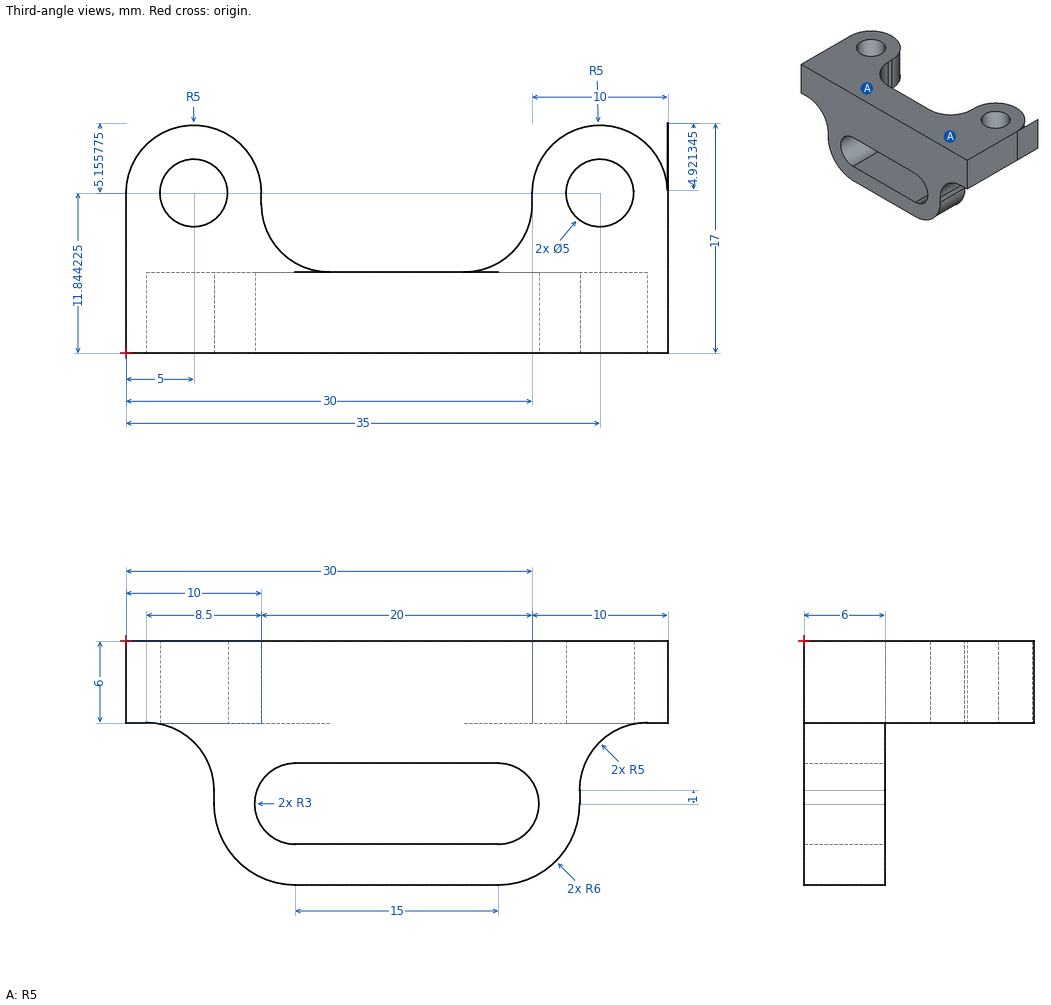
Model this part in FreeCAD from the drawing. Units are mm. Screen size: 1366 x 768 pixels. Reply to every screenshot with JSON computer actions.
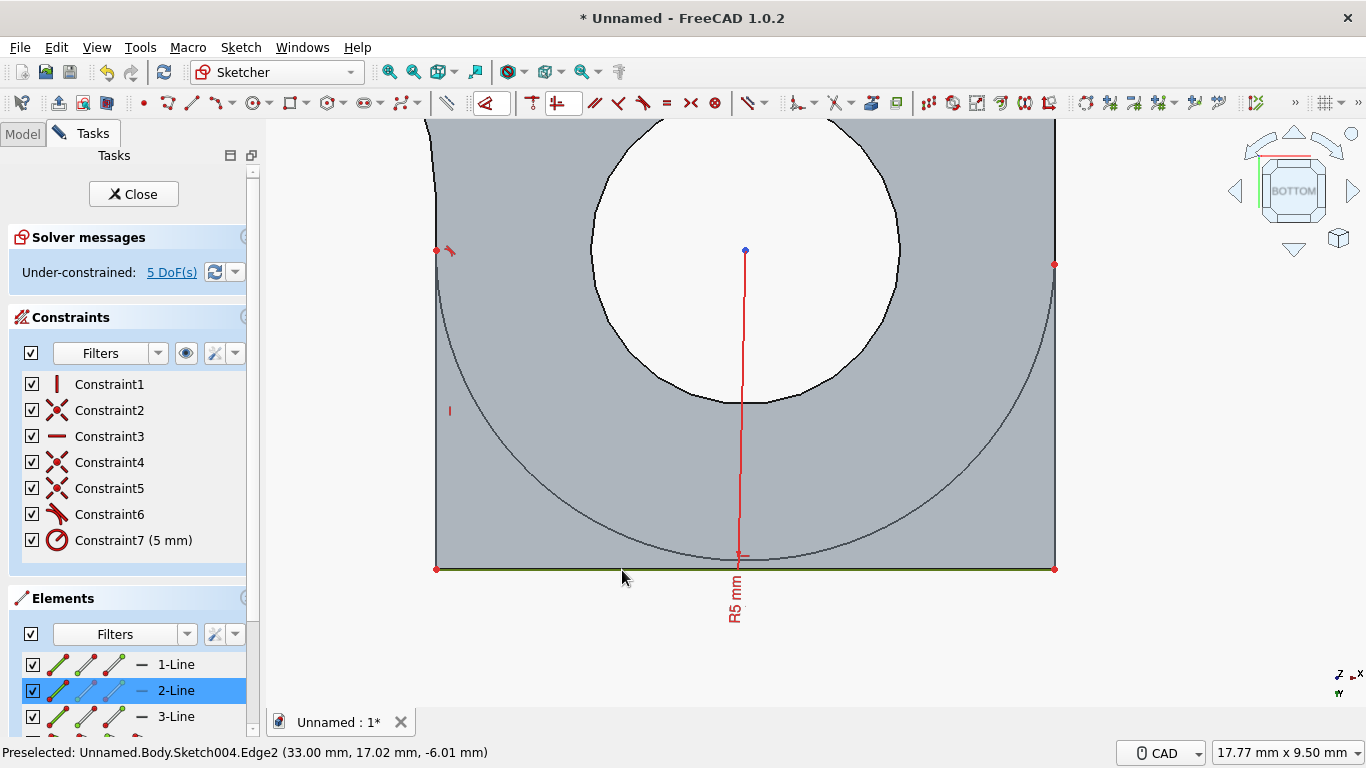
{"action": "key", "text": "l"}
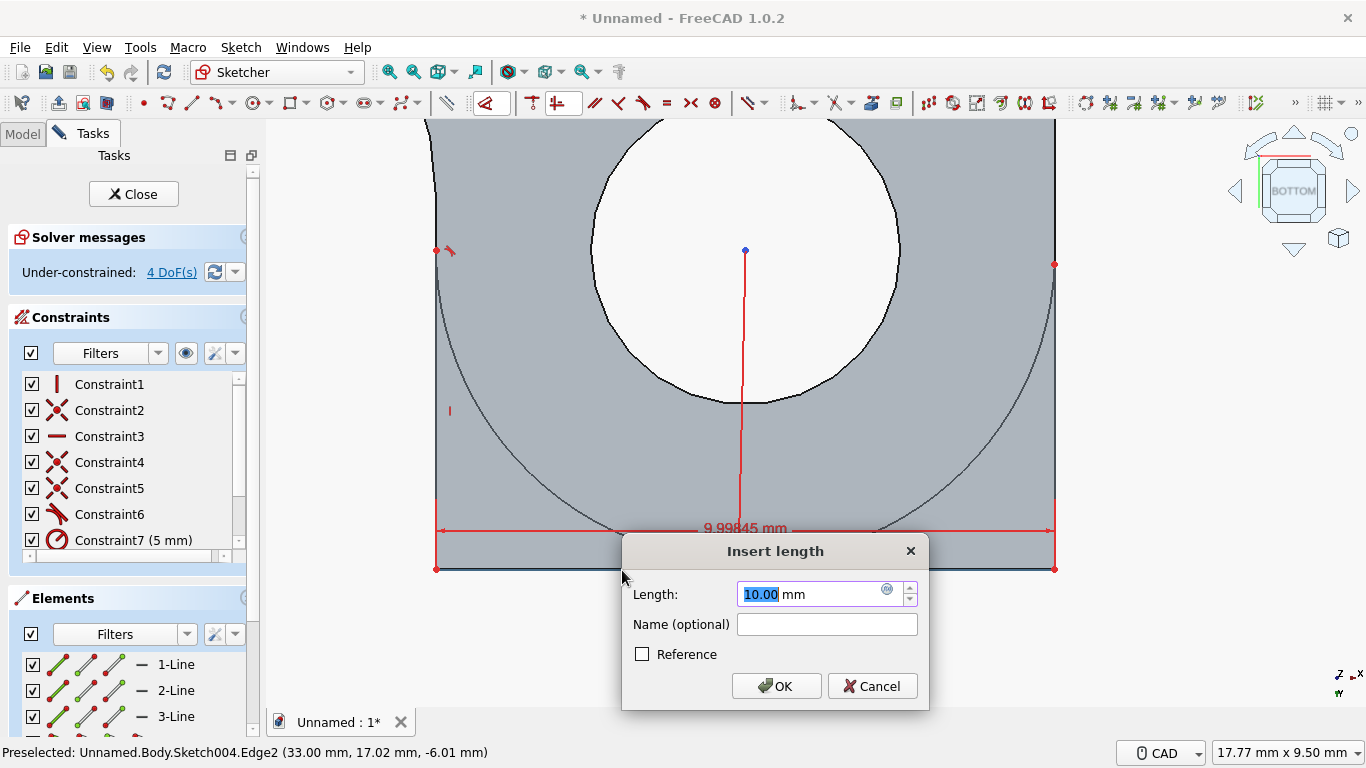
{"action": "type", "text": "10"}
{"action": "key", "text": "Return"}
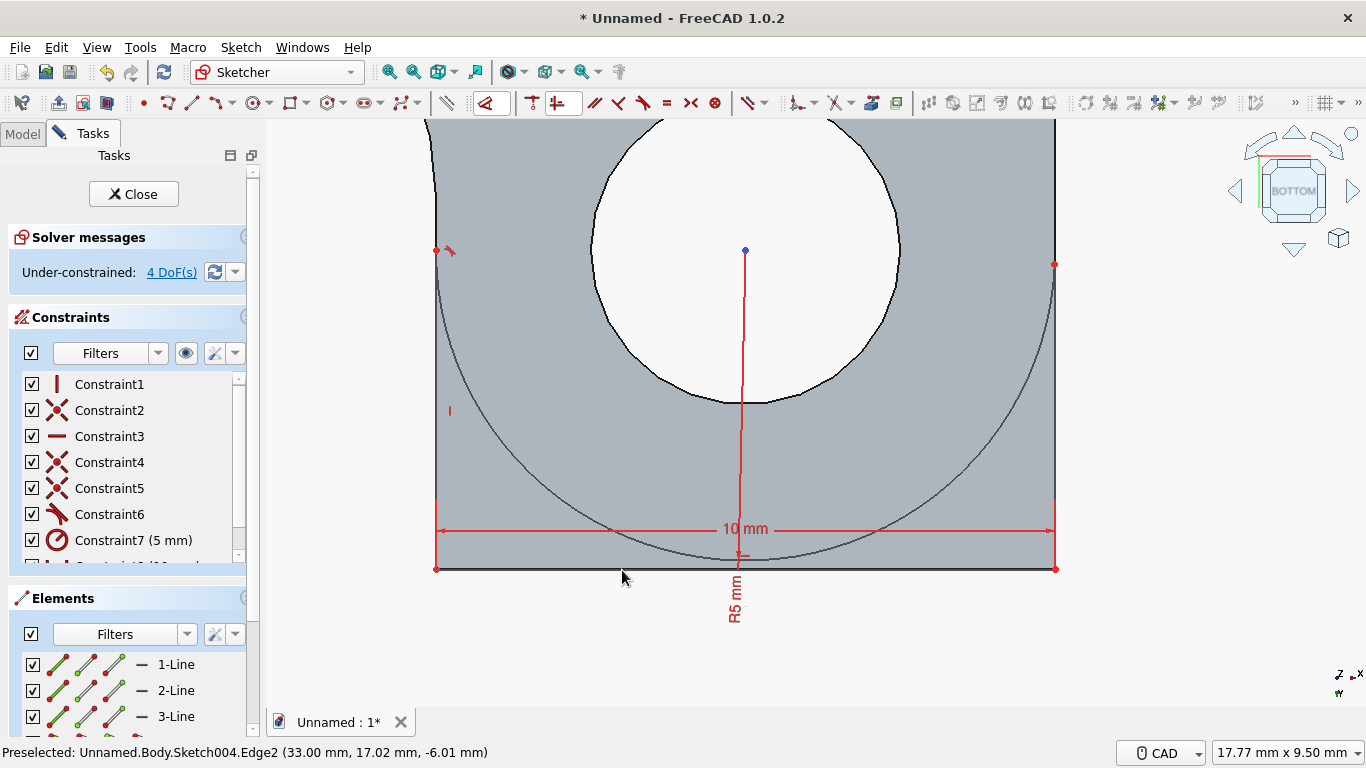
{"action": "left_click", "coordinate": [436, 251]}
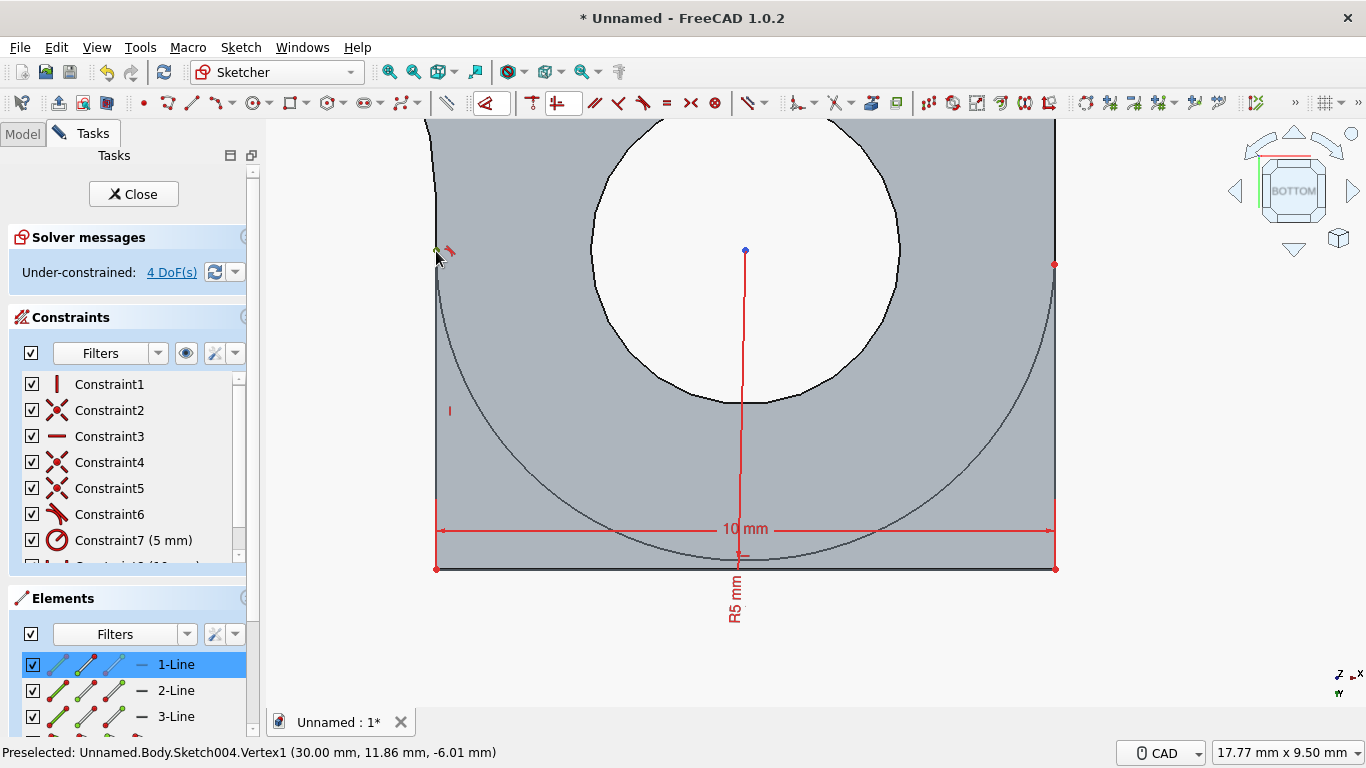
{"action": "key", "text": "l"}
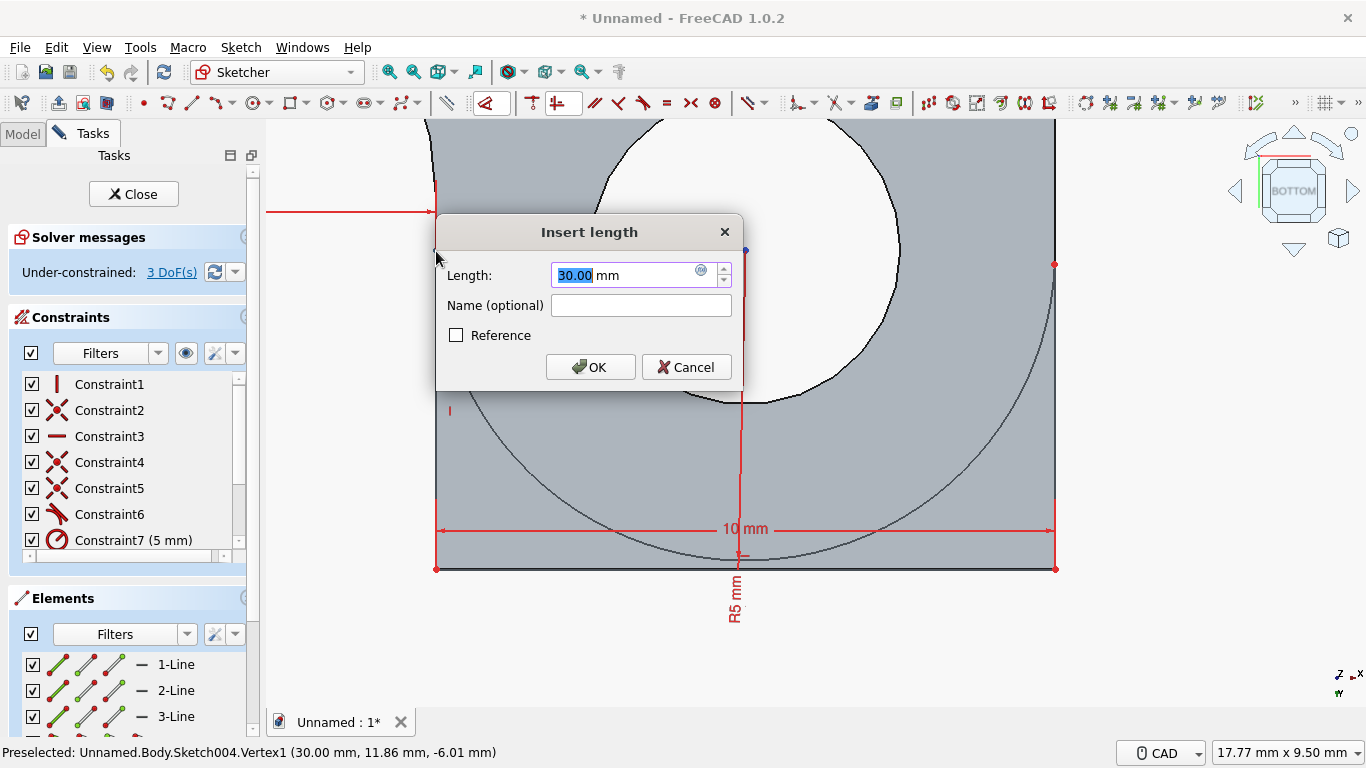
{"action": "type", "text": "30"}
{"action": "key", "text": "Return"}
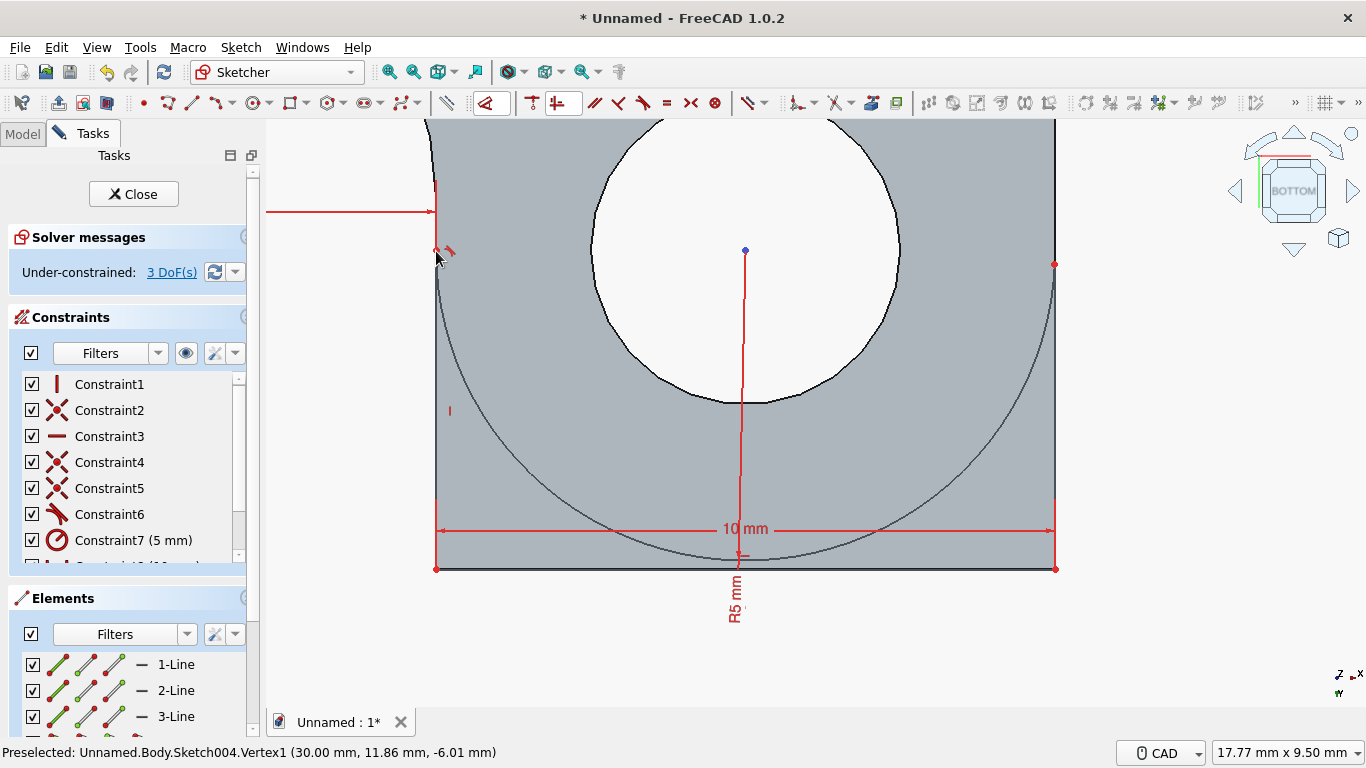
{"action": "left_click", "coordinate": [436, 570]}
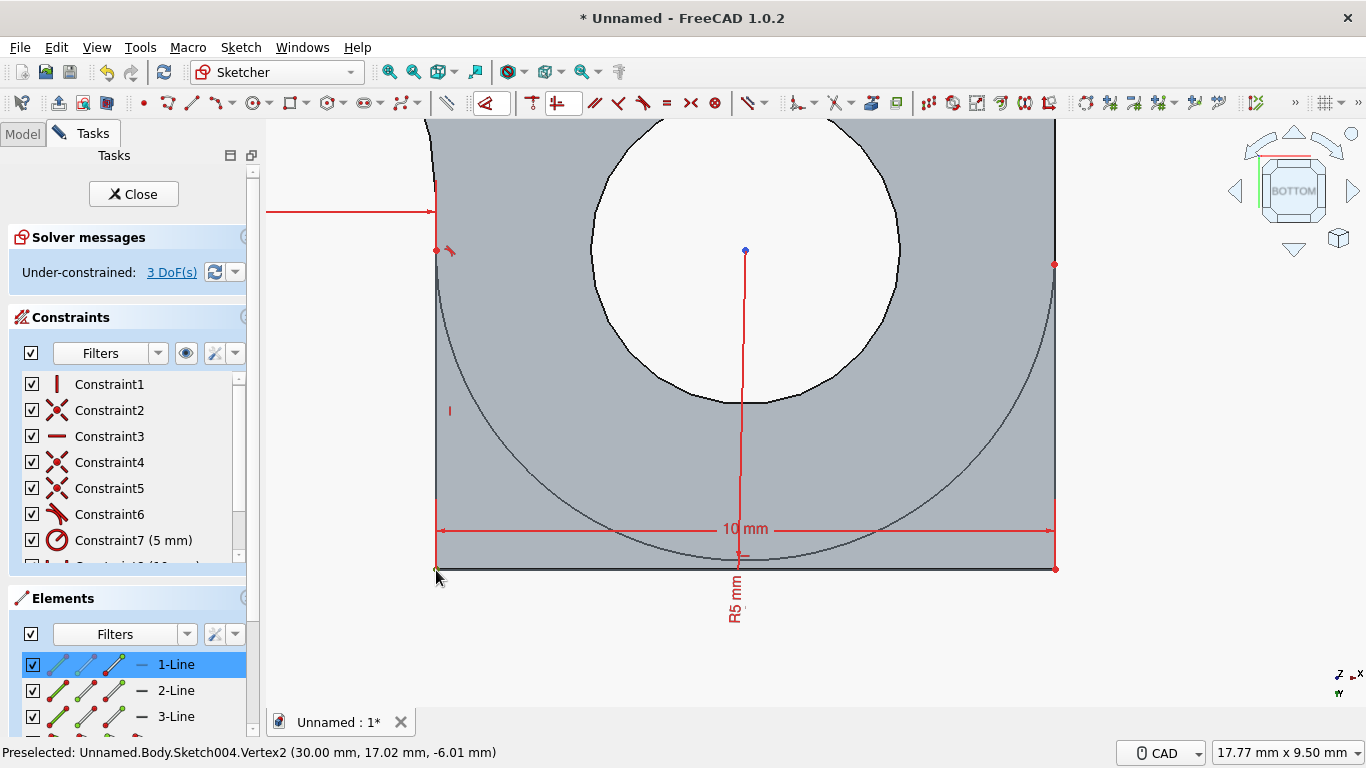
{"action": "left_click", "coordinate": [504, 104]}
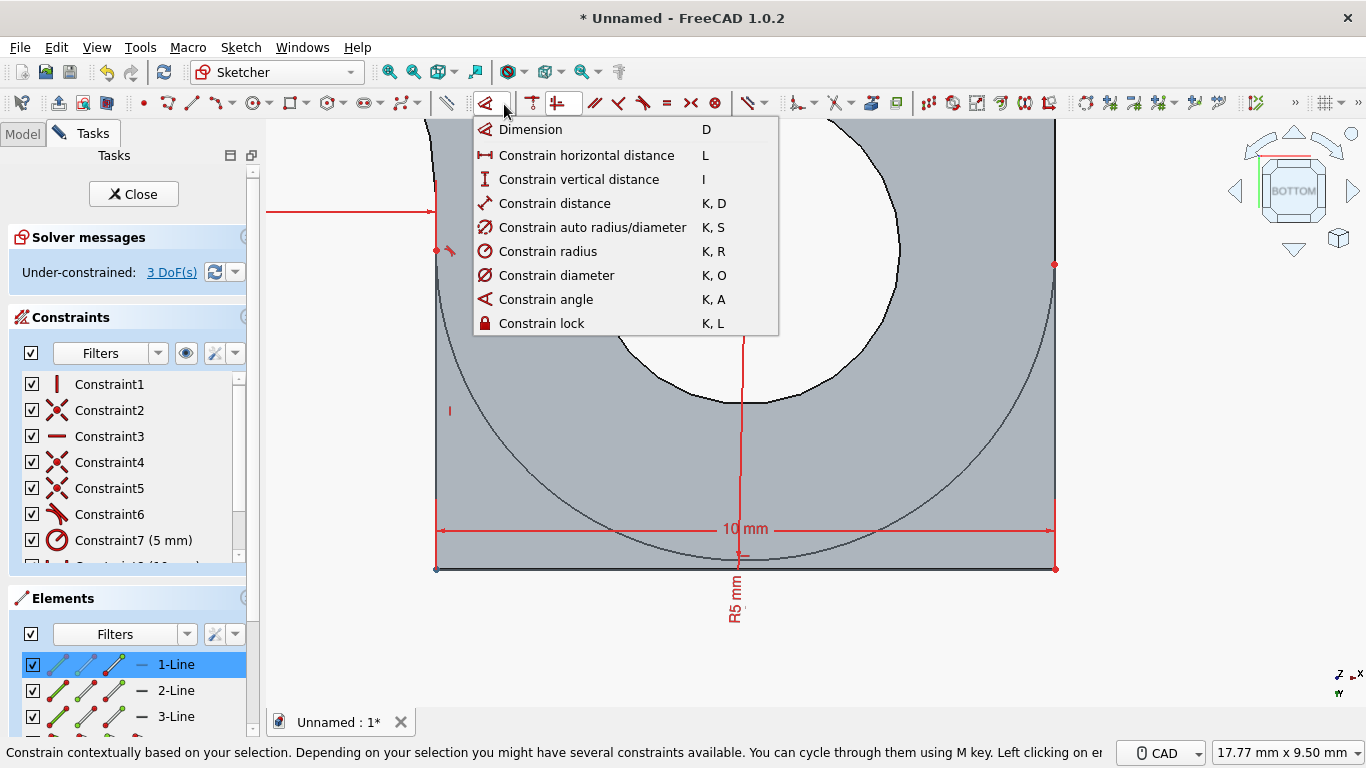
{"action": "left_click", "coordinate": [626, 179]}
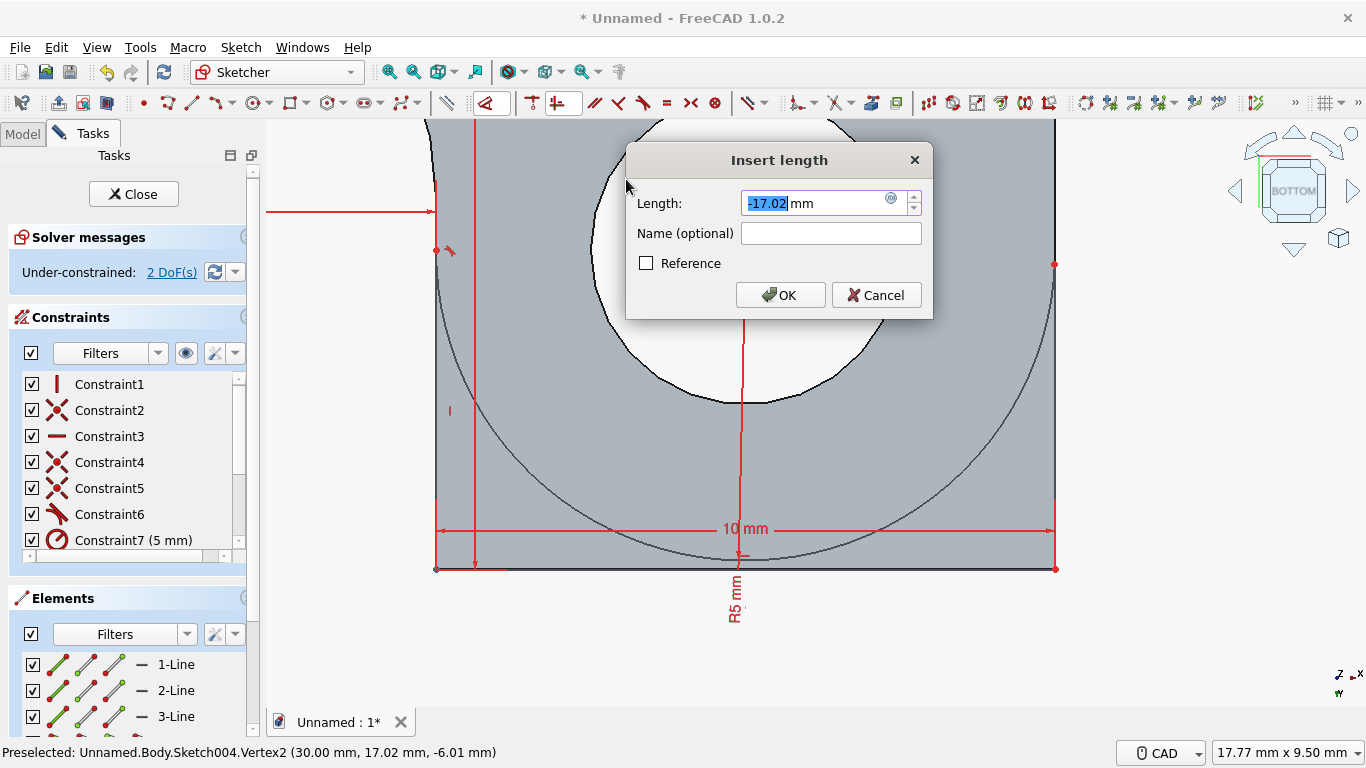
{"action": "type", "text": "-17"}
{"action": "key", "text": "Return"}